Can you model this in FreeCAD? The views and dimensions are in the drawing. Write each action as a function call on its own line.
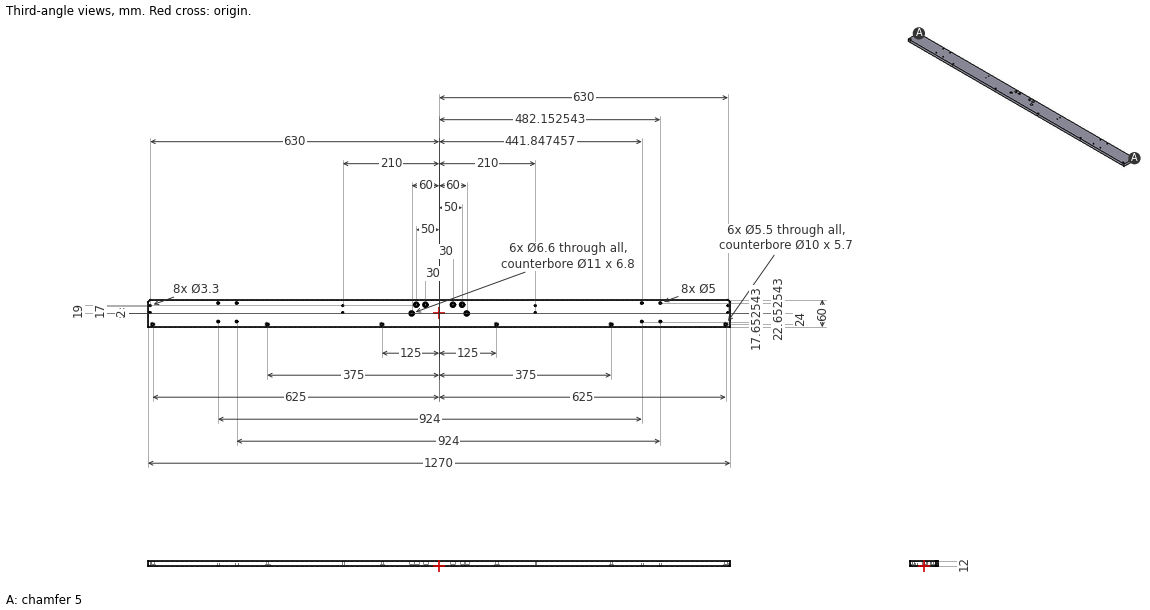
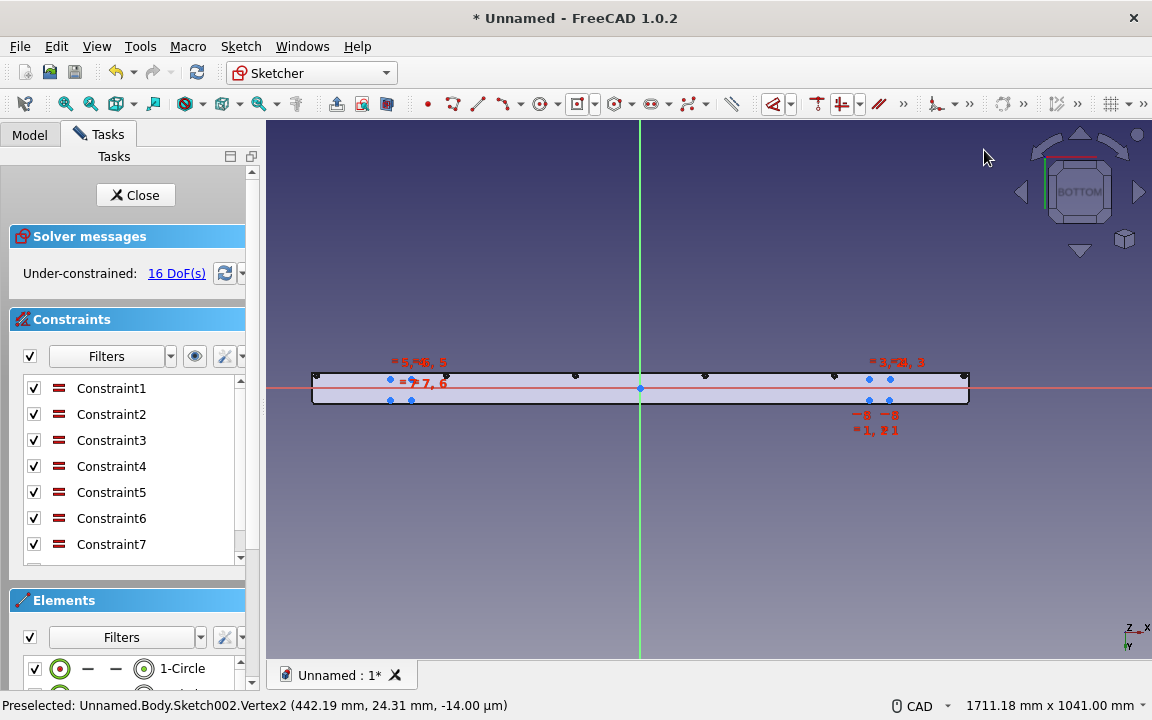
click(869, 401)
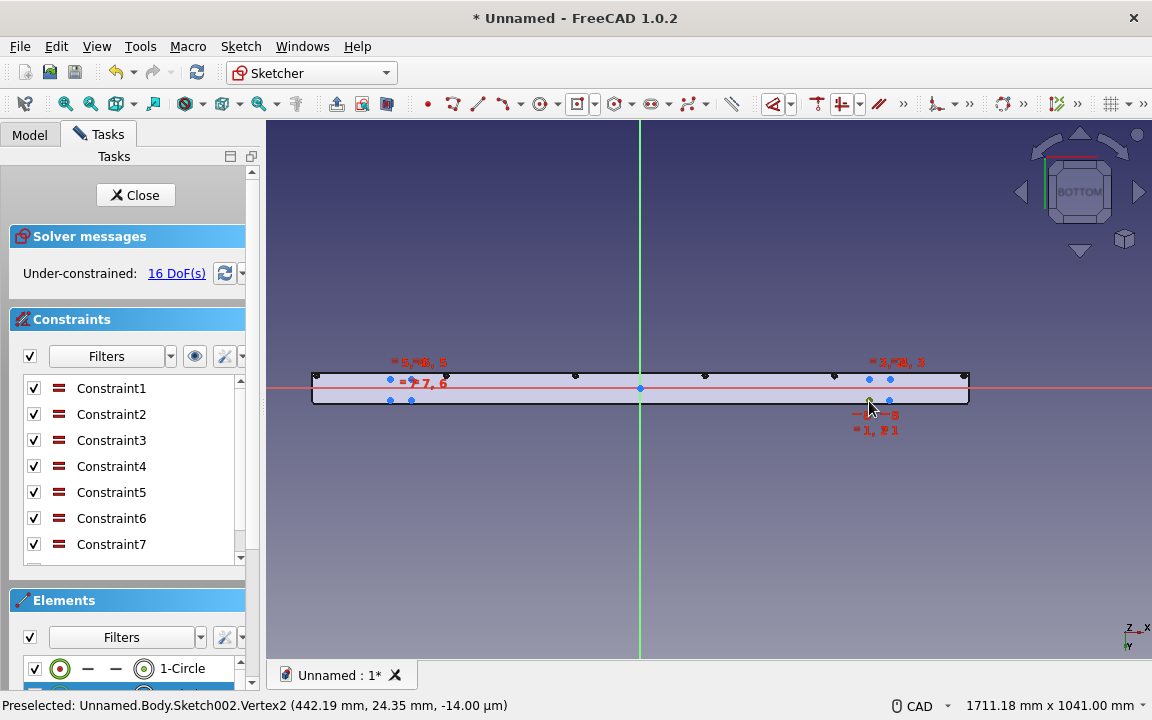
click(869, 380)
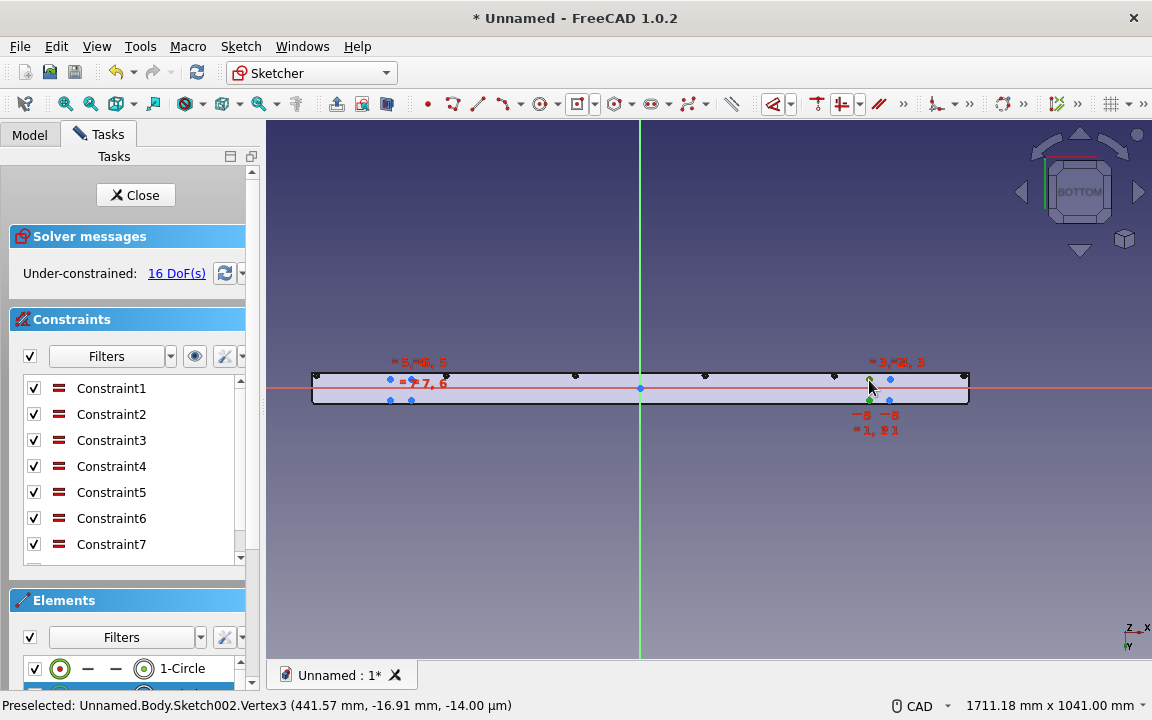
key(v)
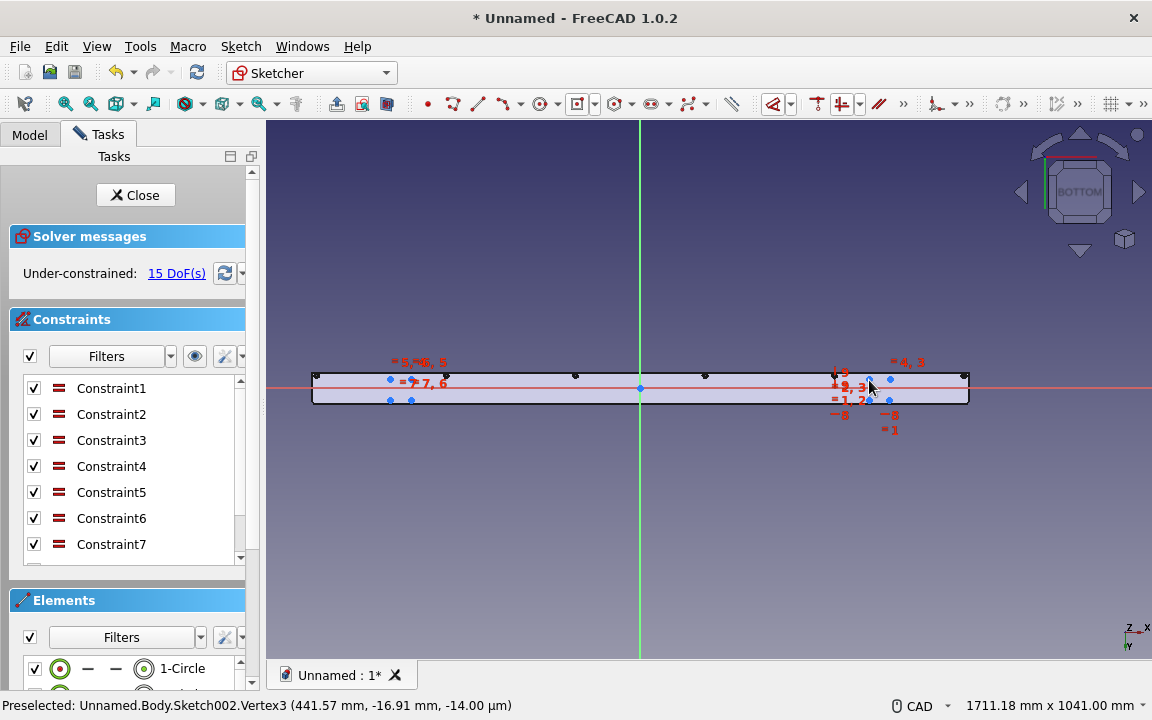
click(890, 401)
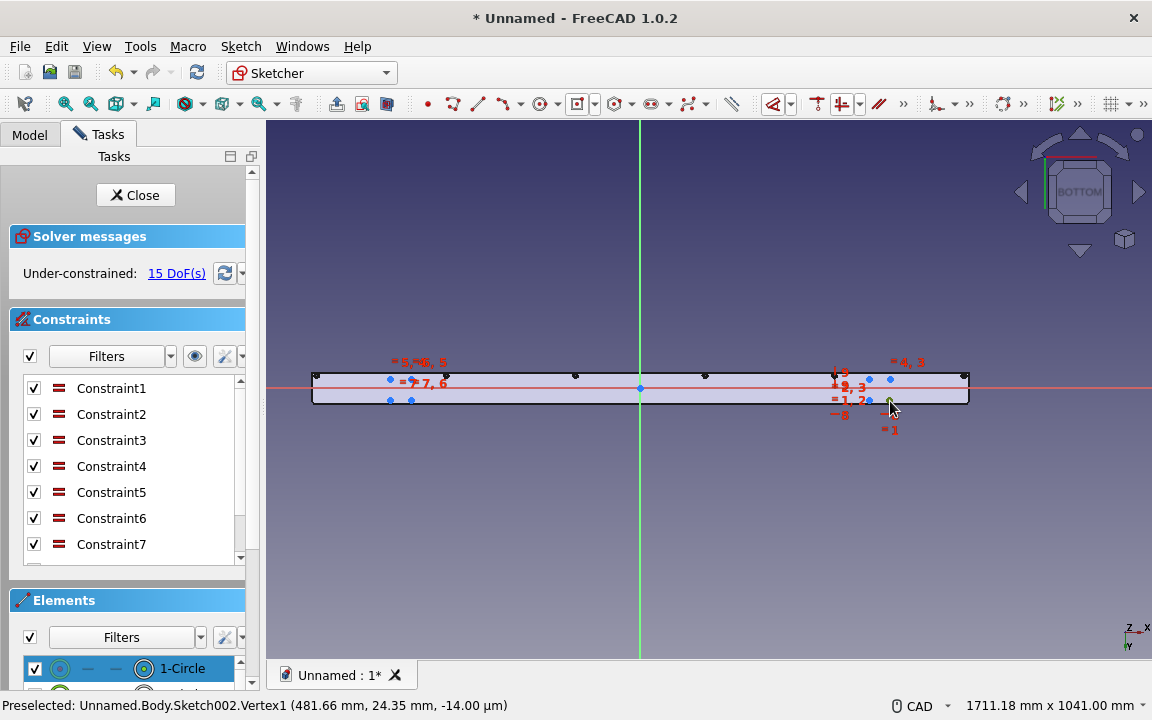
click(890, 380)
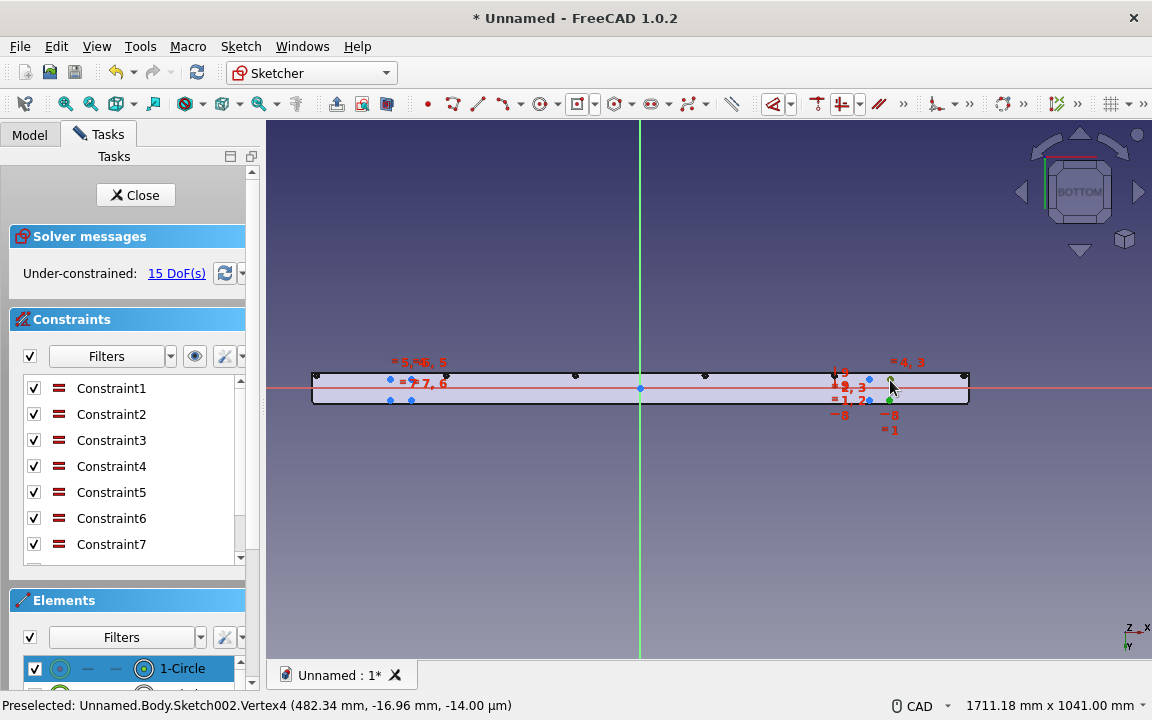
key(v)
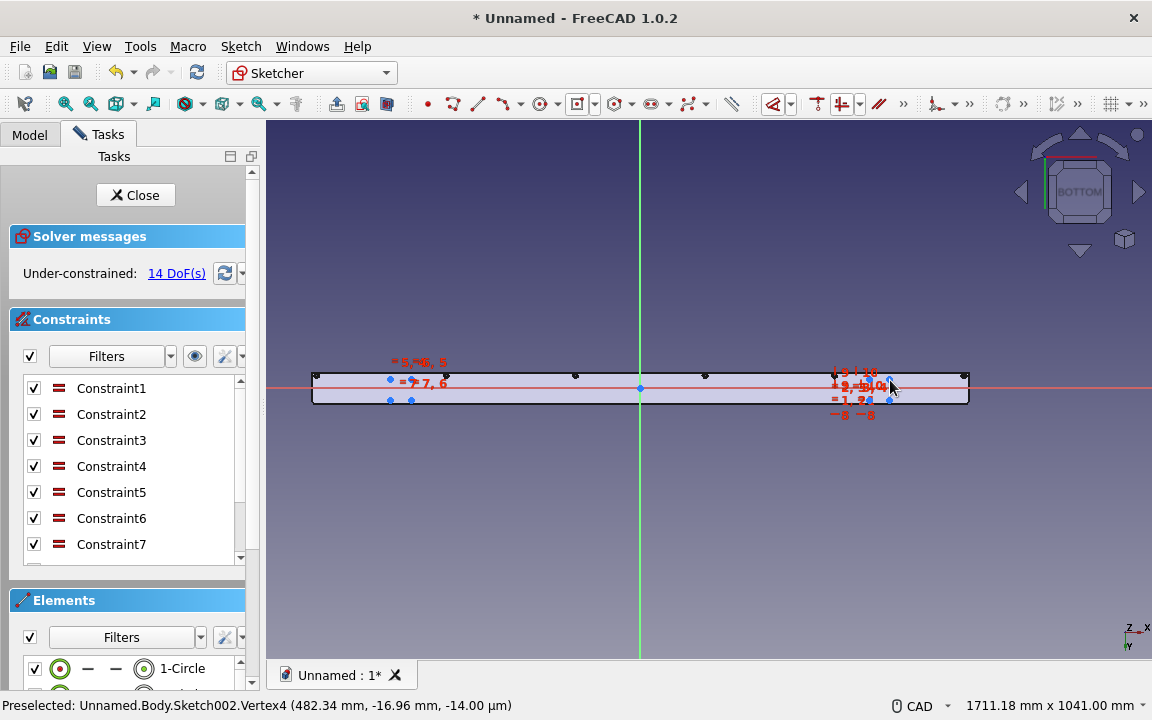
scroll(869, 380, up, 4)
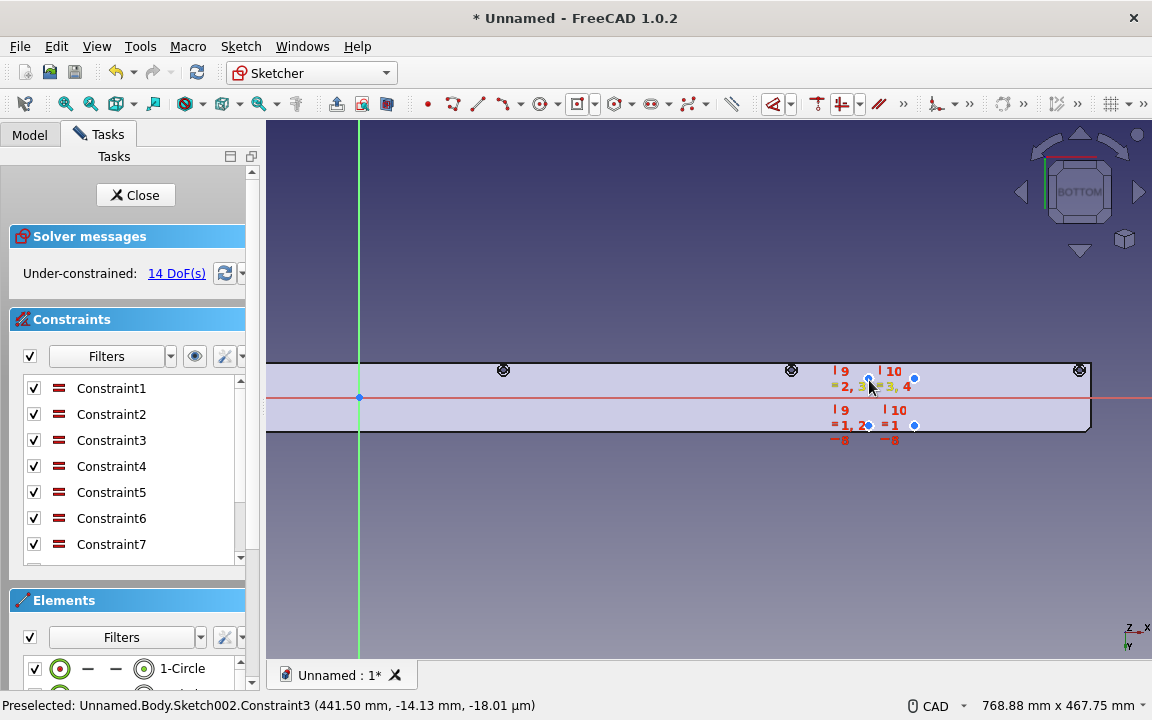
click(869, 378)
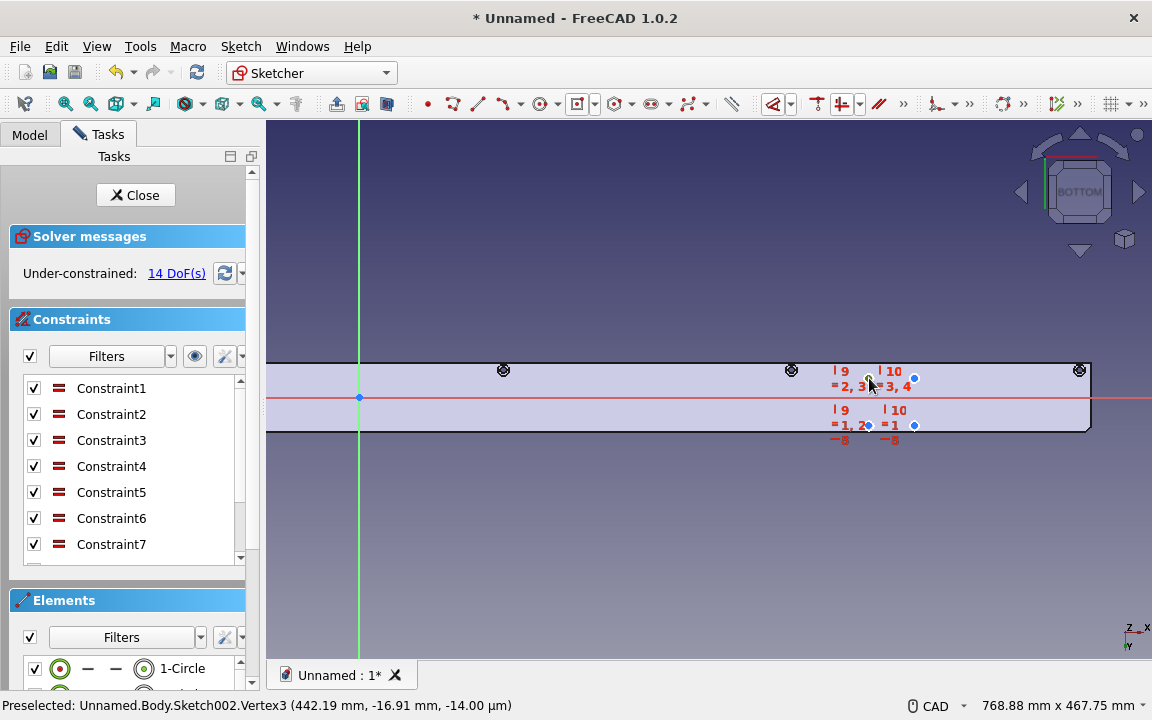
click(914, 378)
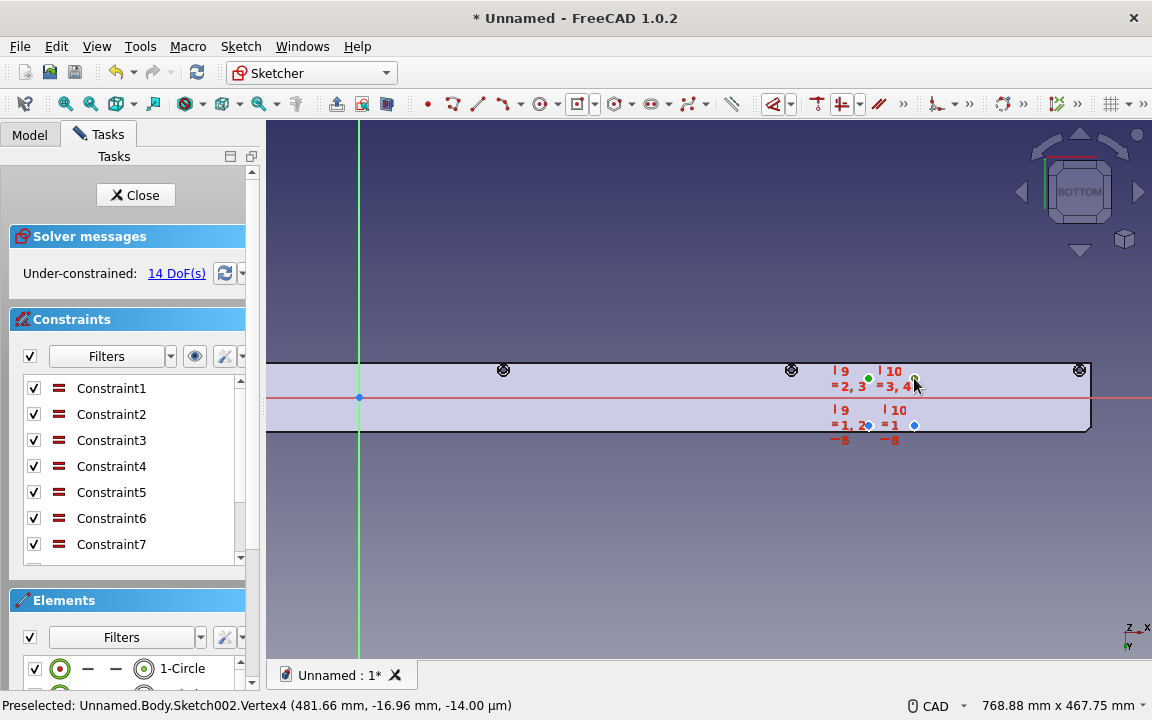
click(860, 104)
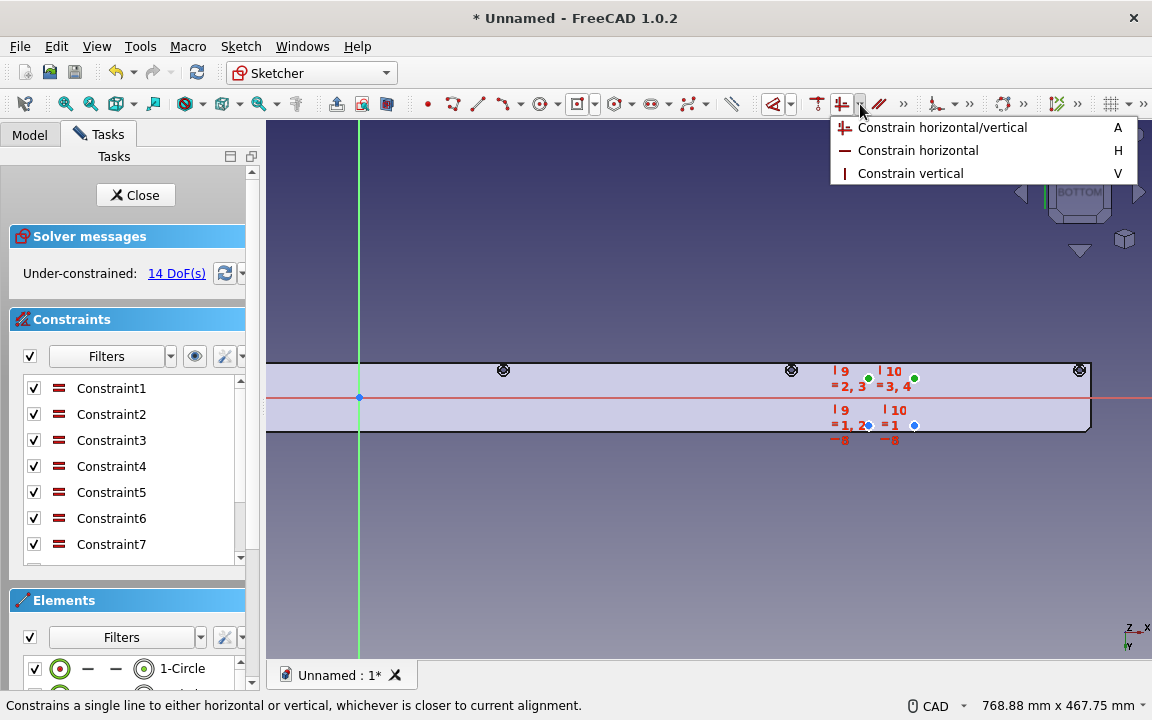
click(984, 150)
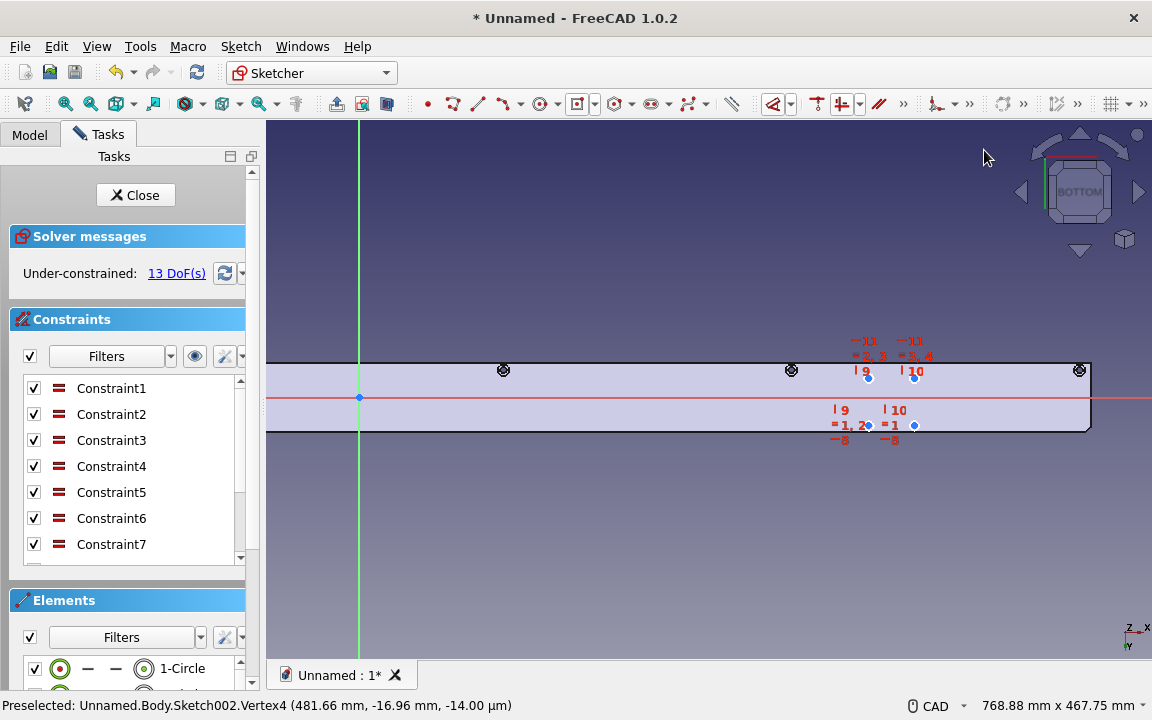
click(869, 378)